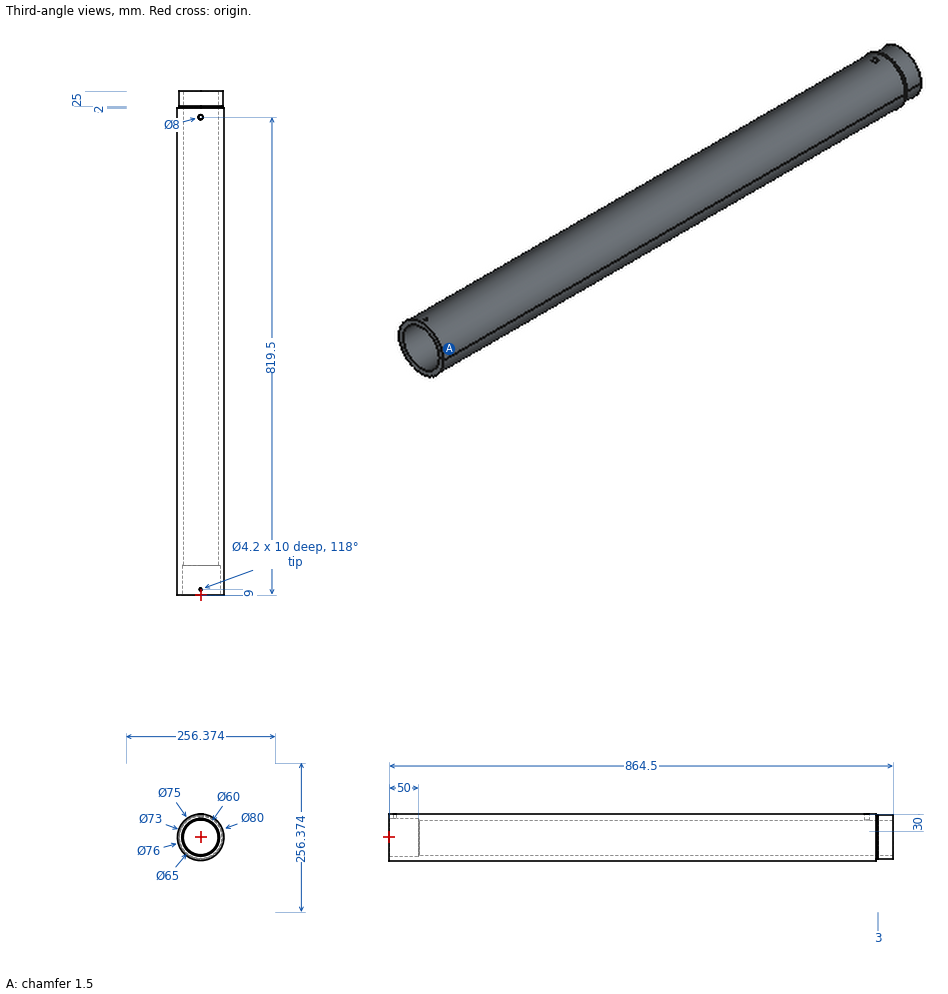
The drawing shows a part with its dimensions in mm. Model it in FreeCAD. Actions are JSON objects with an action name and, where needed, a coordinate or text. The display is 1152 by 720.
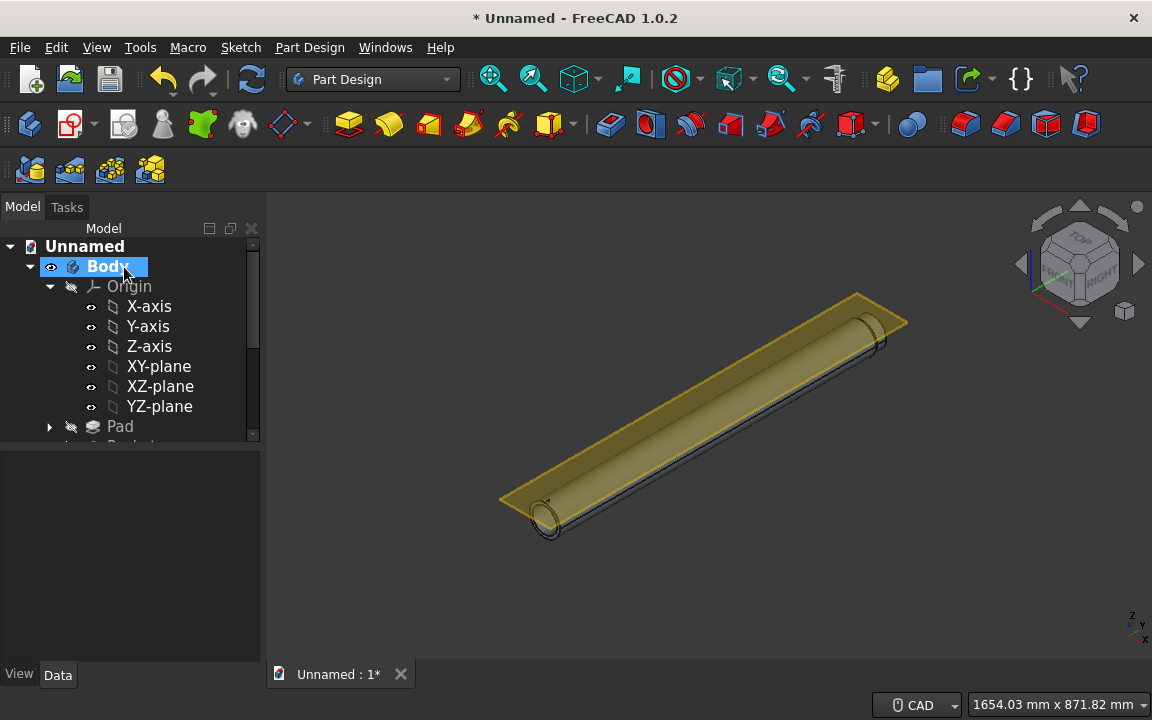
{"action": "scroll", "coordinate": [100, 342], "scroll_direction": "down", "scroll_amount": 3}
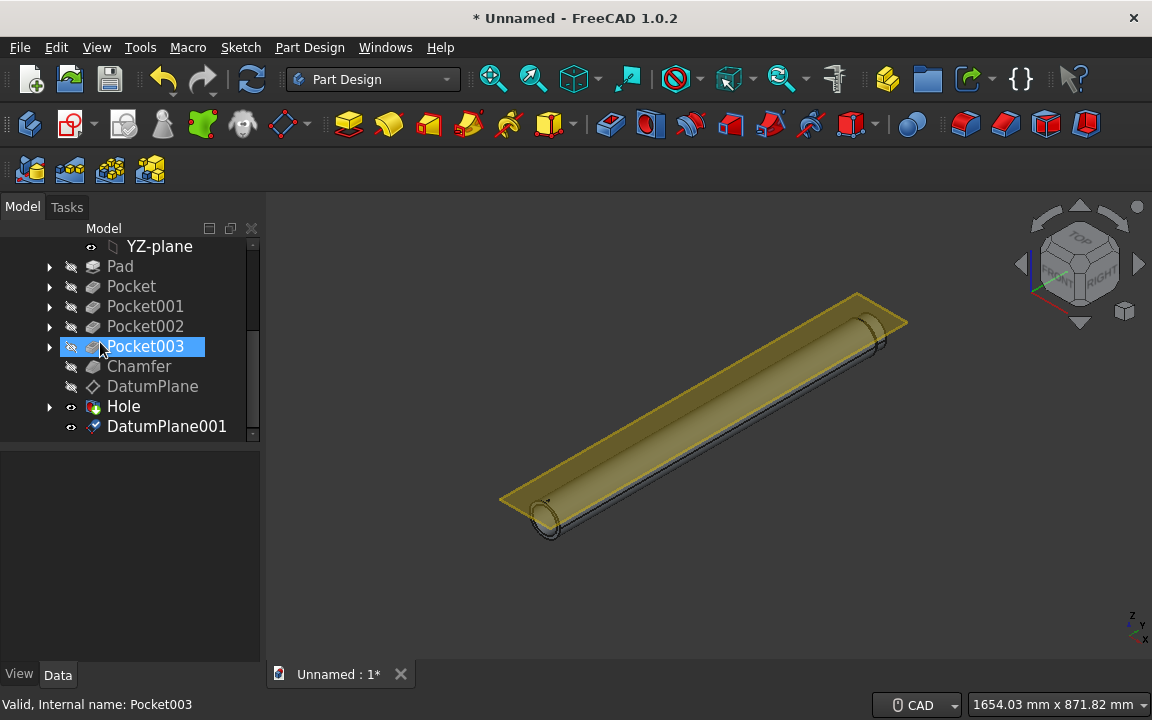
{"action": "left_click", "coordinate": [116, 427]}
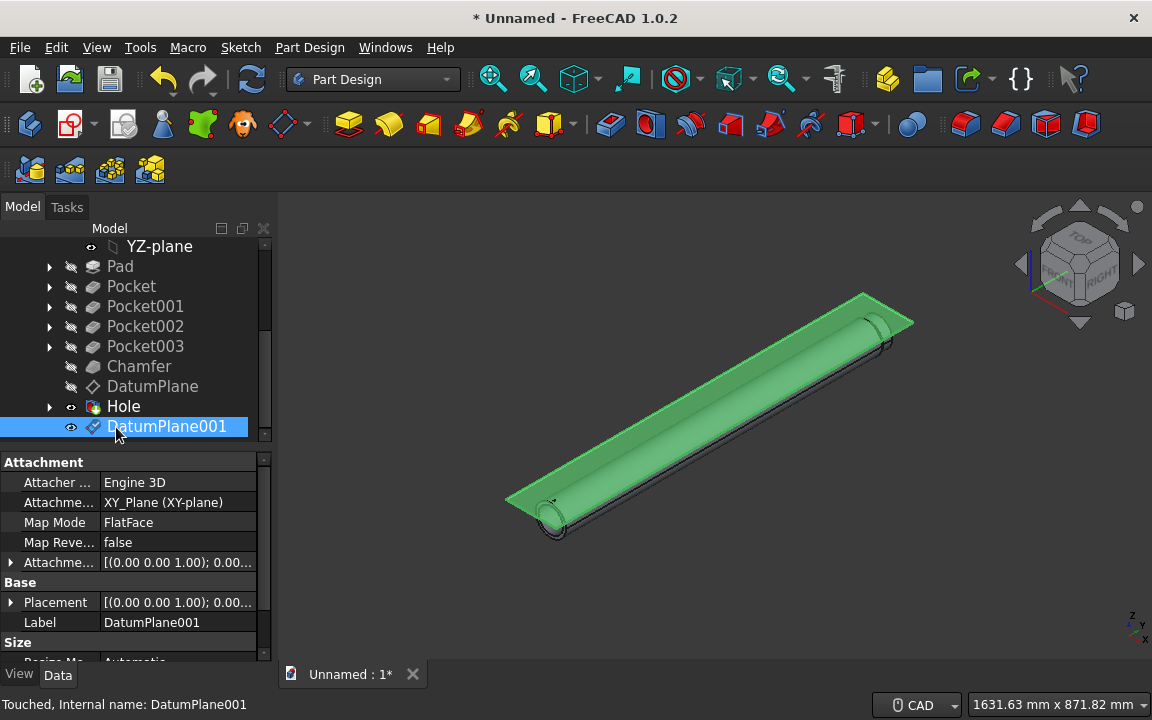
{"action": "left_click", "coordinate": [70, 124]}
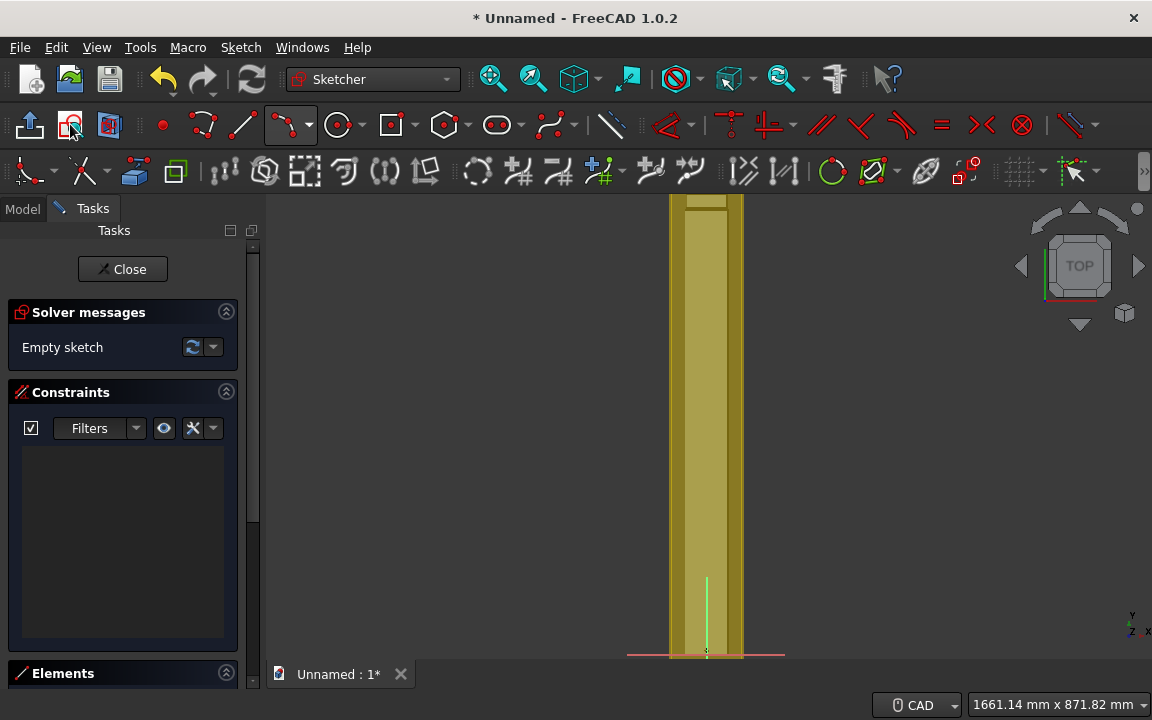
{"action": "scroll", "coordinate": [640, 426], "scroll_direction": "down", "scroll_amount": 5}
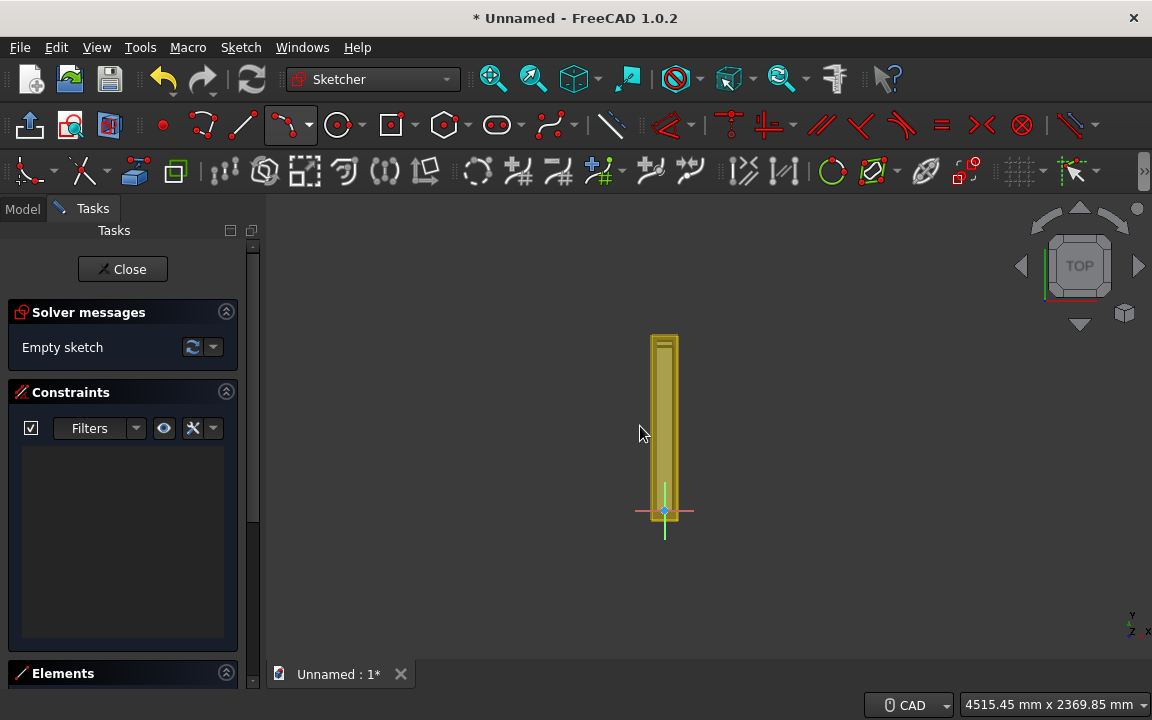
{"action": "scroll", "coordinate": [666, 346], "scroll_direction": "up", "scroll_amount": 15}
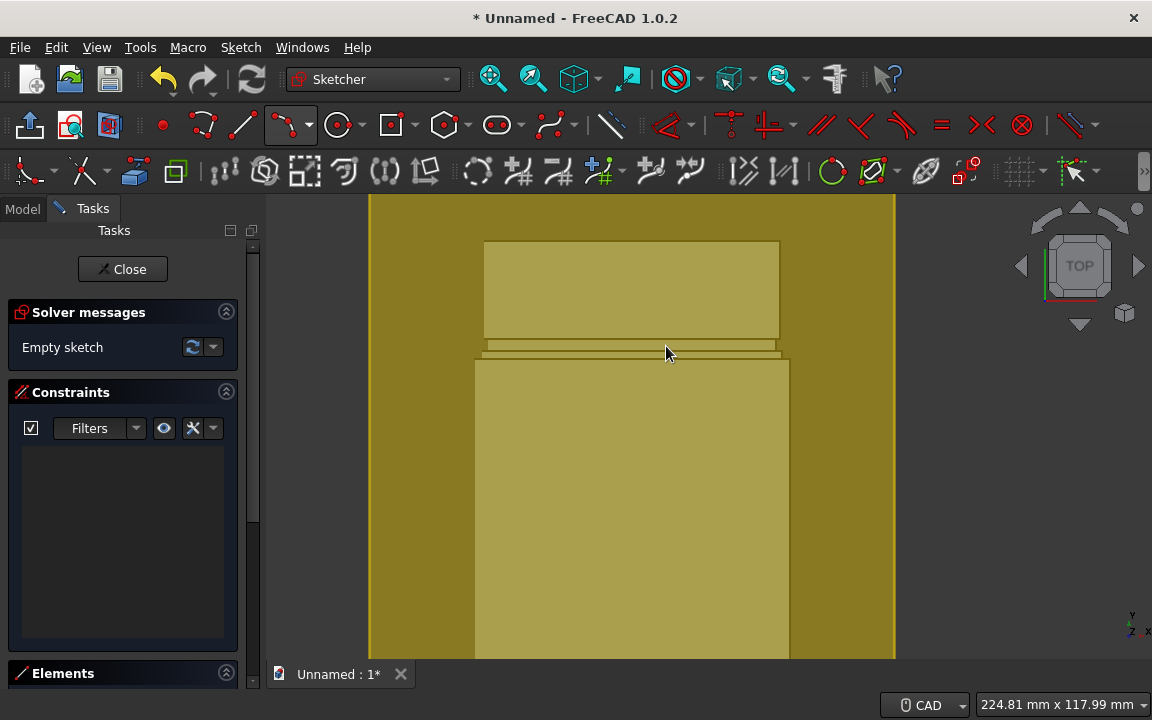
{"action": "scroll", "coordinate": [631, 417], "scroll_direction": "up", "scroll_amount": 11}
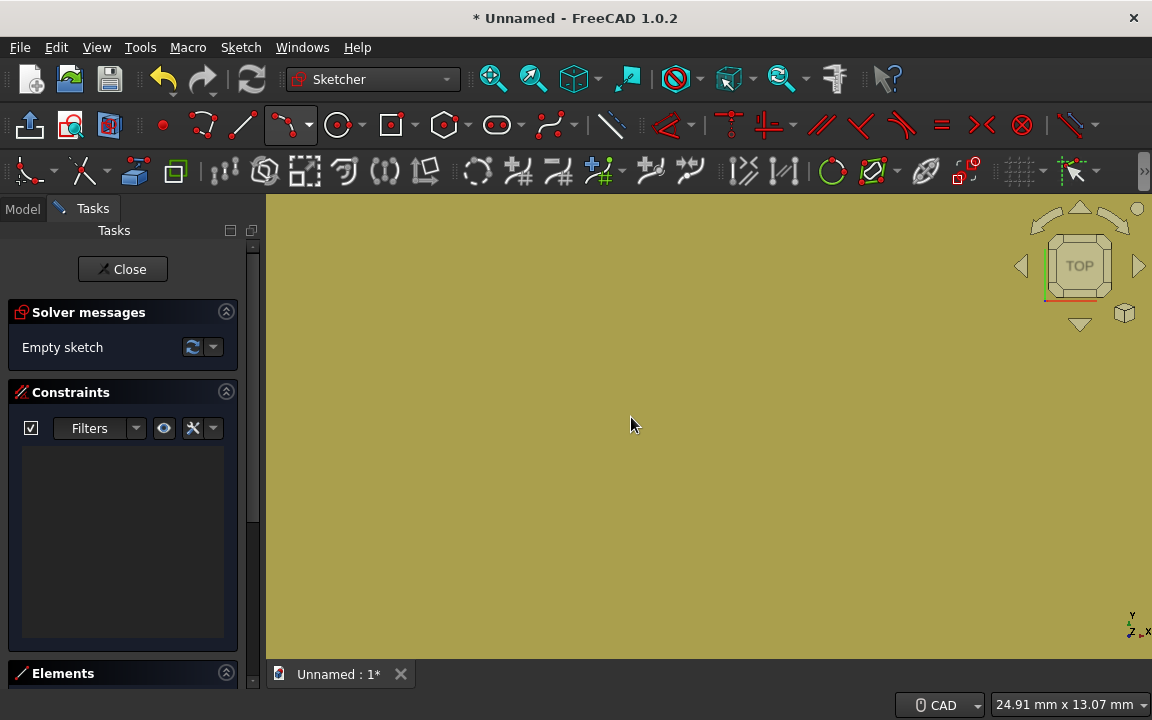
{"action": "key", "text": "g c"}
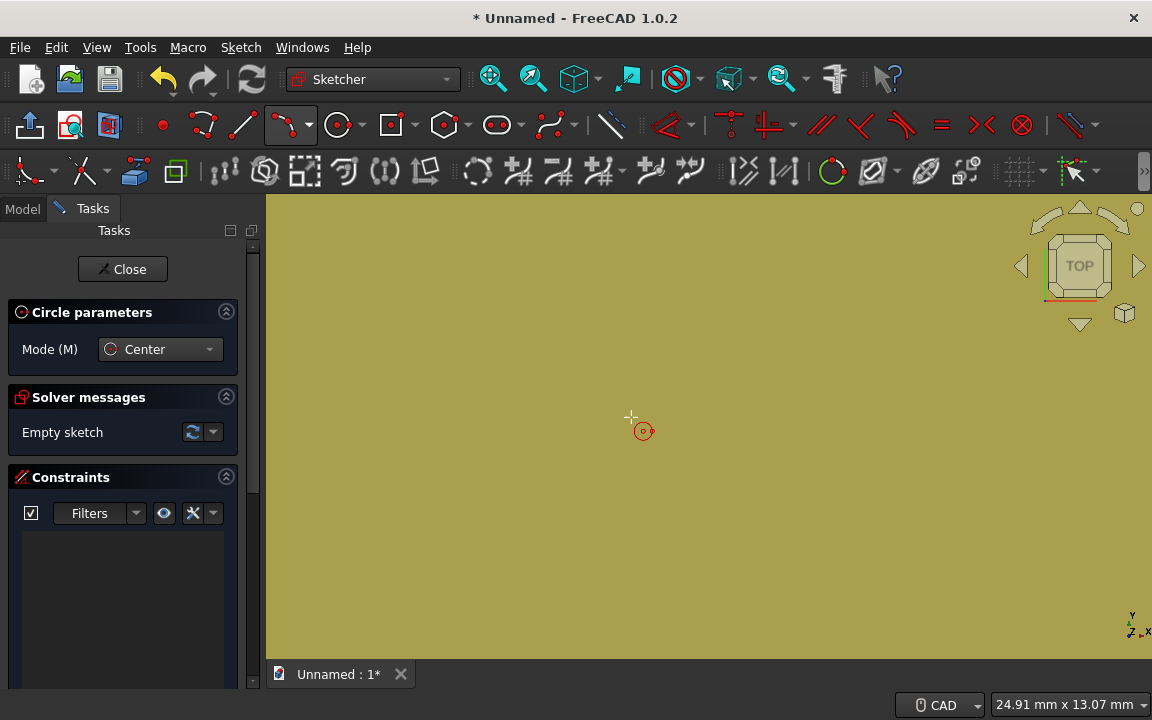
{"action": "left_click", "coordinate": [638, 421]}
{"action": "mouse_move", "coordinate": [739, 320]}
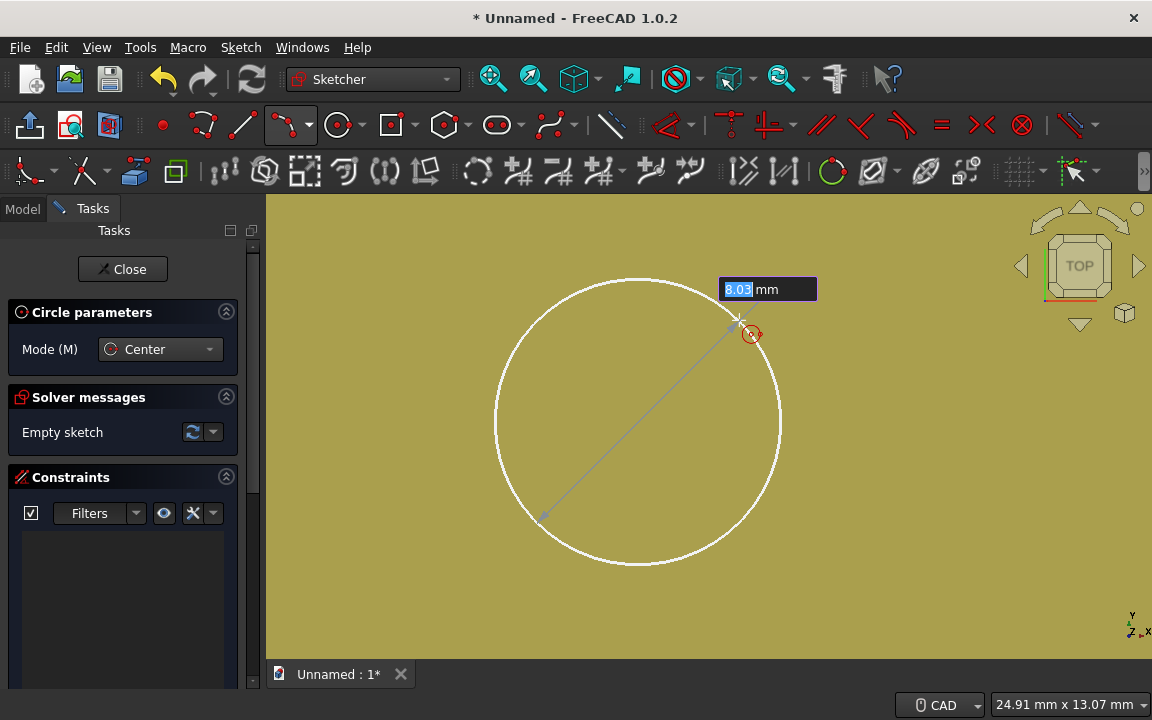
{"action": "type", "text": "8"}
{"action": "key", "text": "Return"}
{"action": "key", "text": "Escape"}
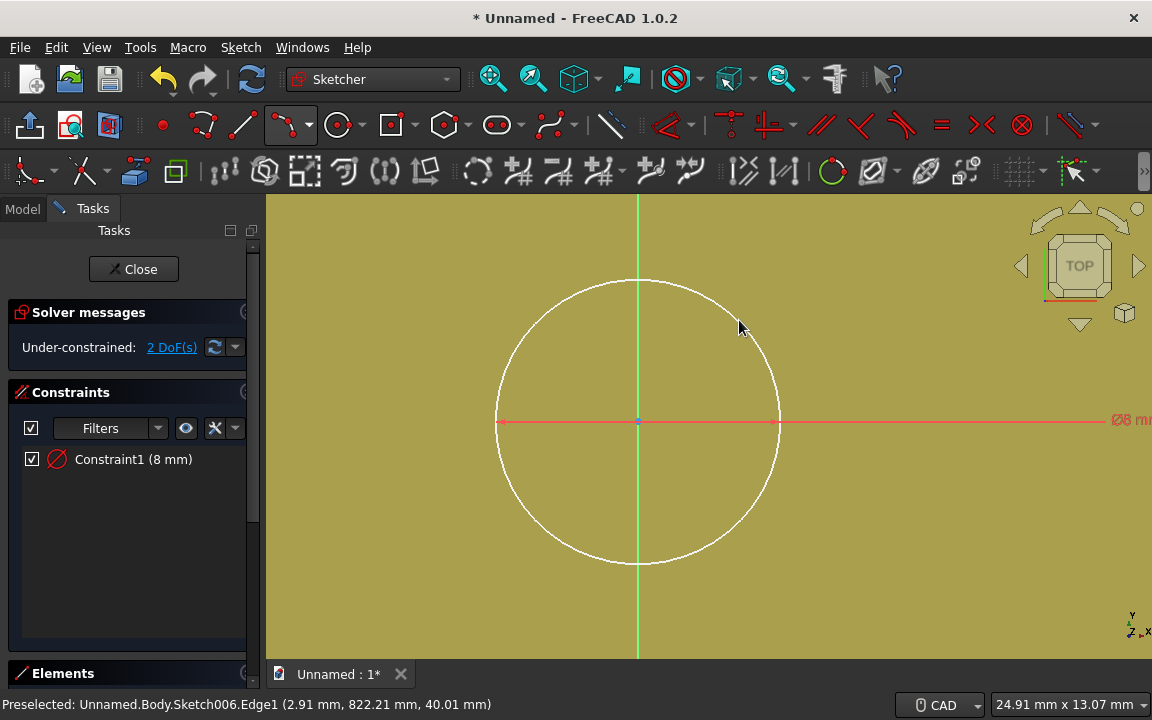
{"action": "left_click", "coordinate": [638, 422]}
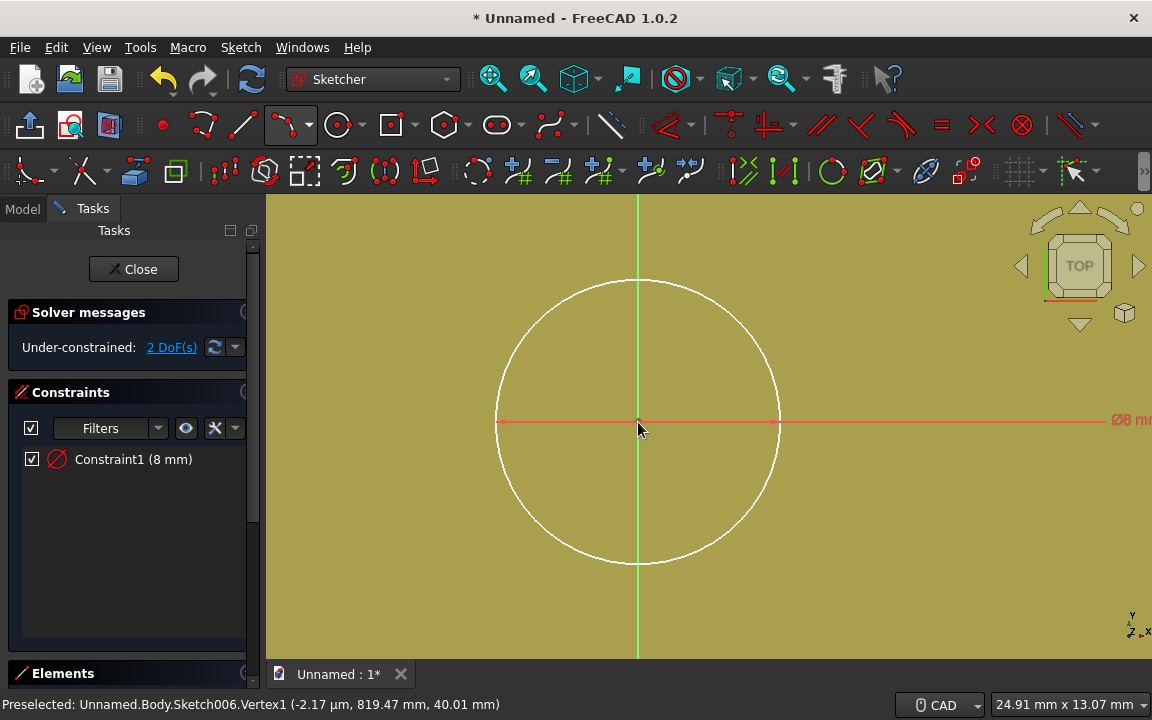
{"action": "left_click", "coordinate": [638, 602]}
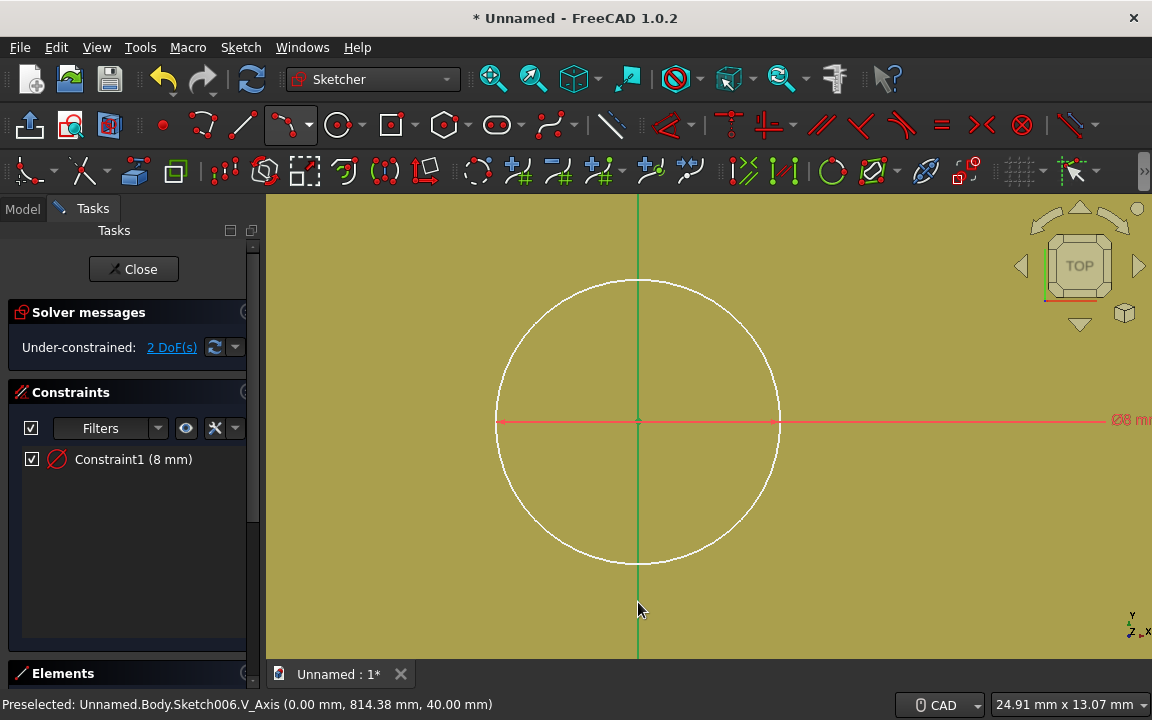
{"action": "left_click", "coordinate": [730, 126]}